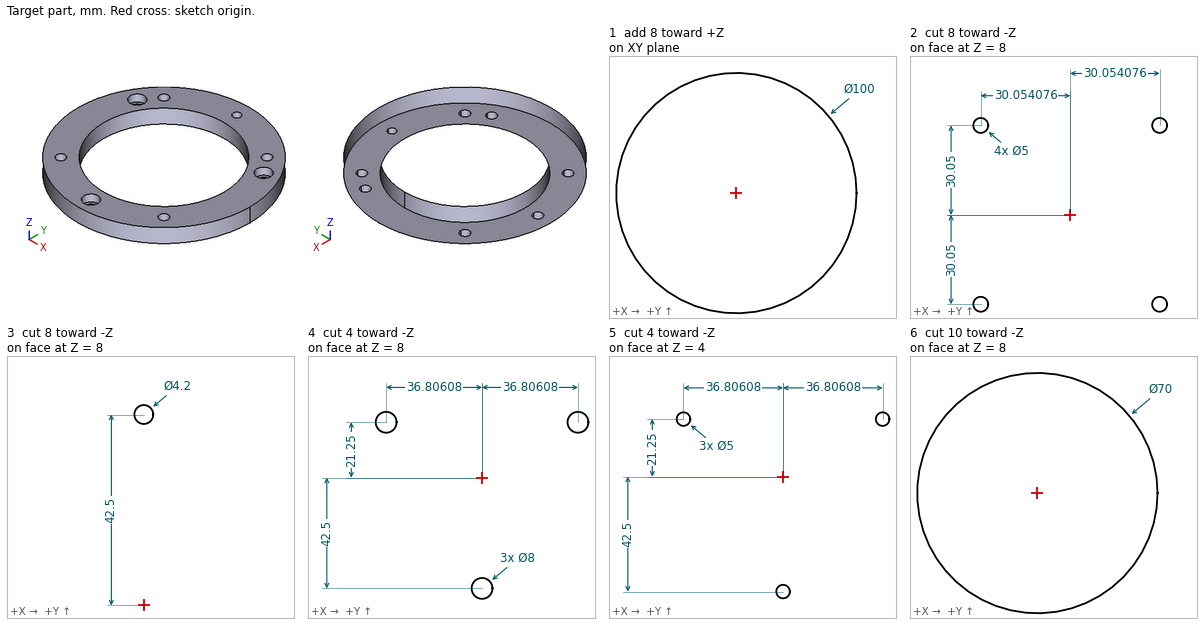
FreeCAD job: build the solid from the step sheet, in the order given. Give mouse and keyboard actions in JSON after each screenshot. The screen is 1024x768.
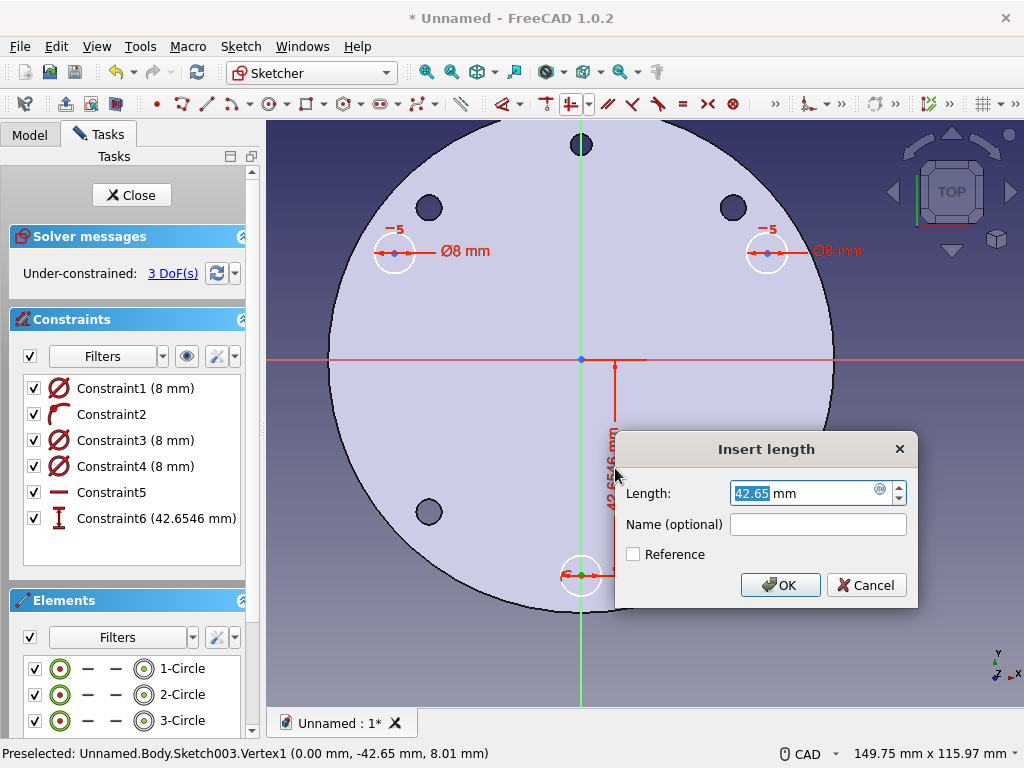
{"action": "type", "text": "42.5"}
{"action": "key", "text": "Return"}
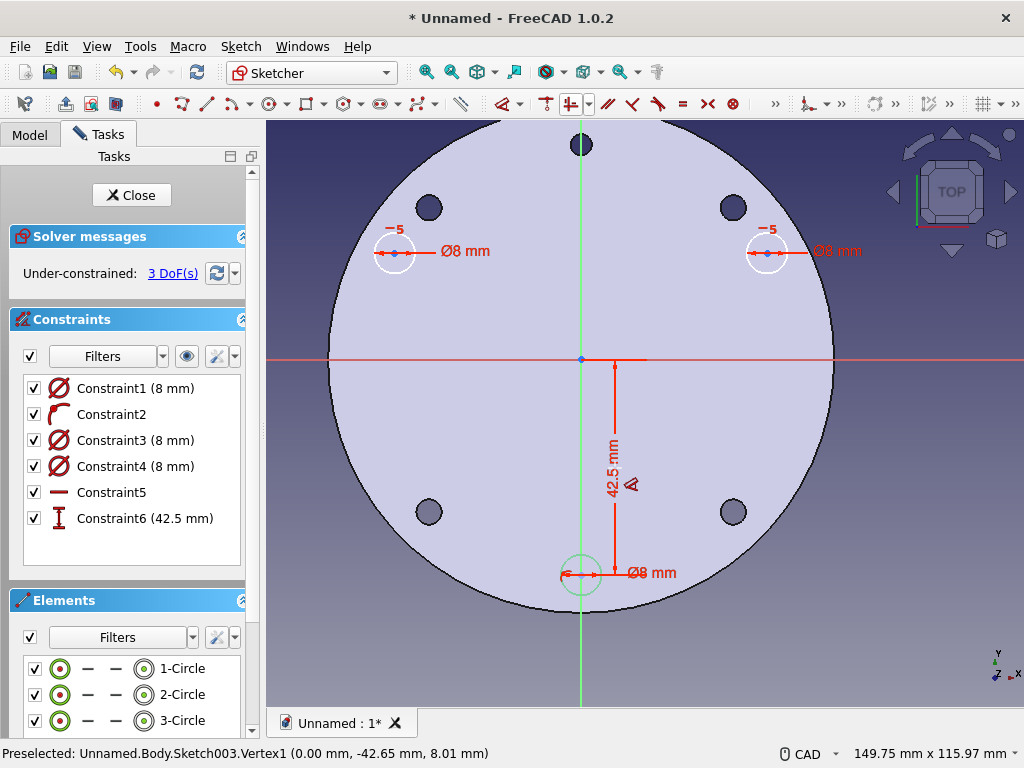
{"action": "left_click", "coordinate": [395, 253]}
{"action": "left_click", "coordinate": [361, 307]}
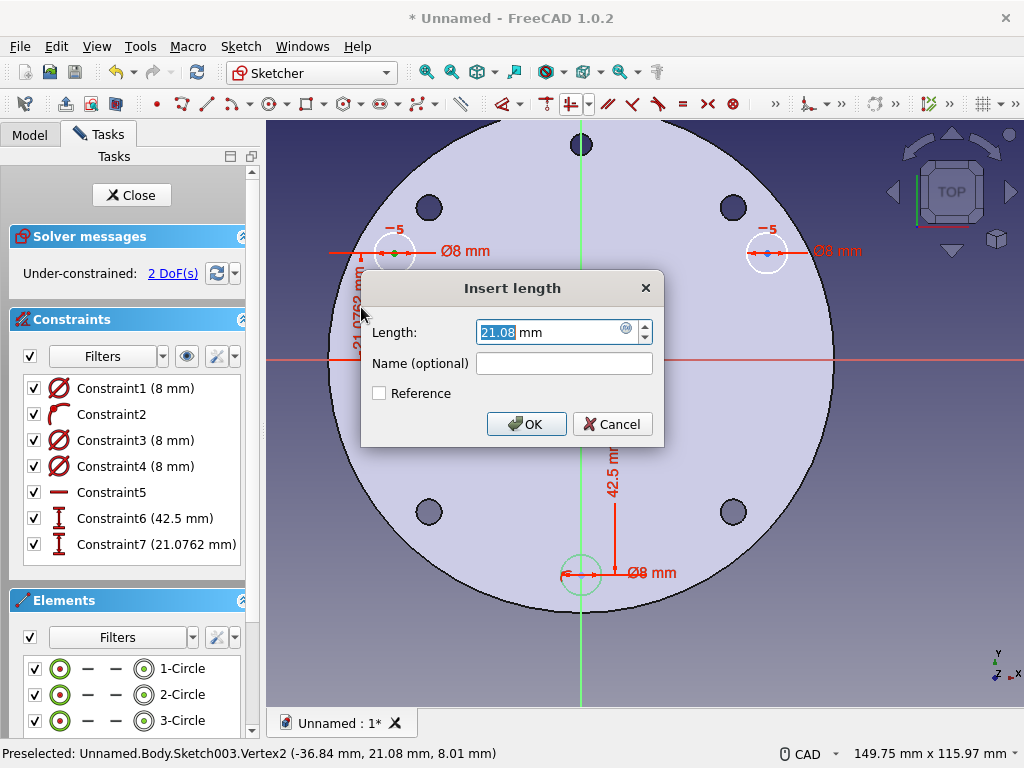
{"action": "type", "text": "21.25"}
{"action": "key", "text": "Return"}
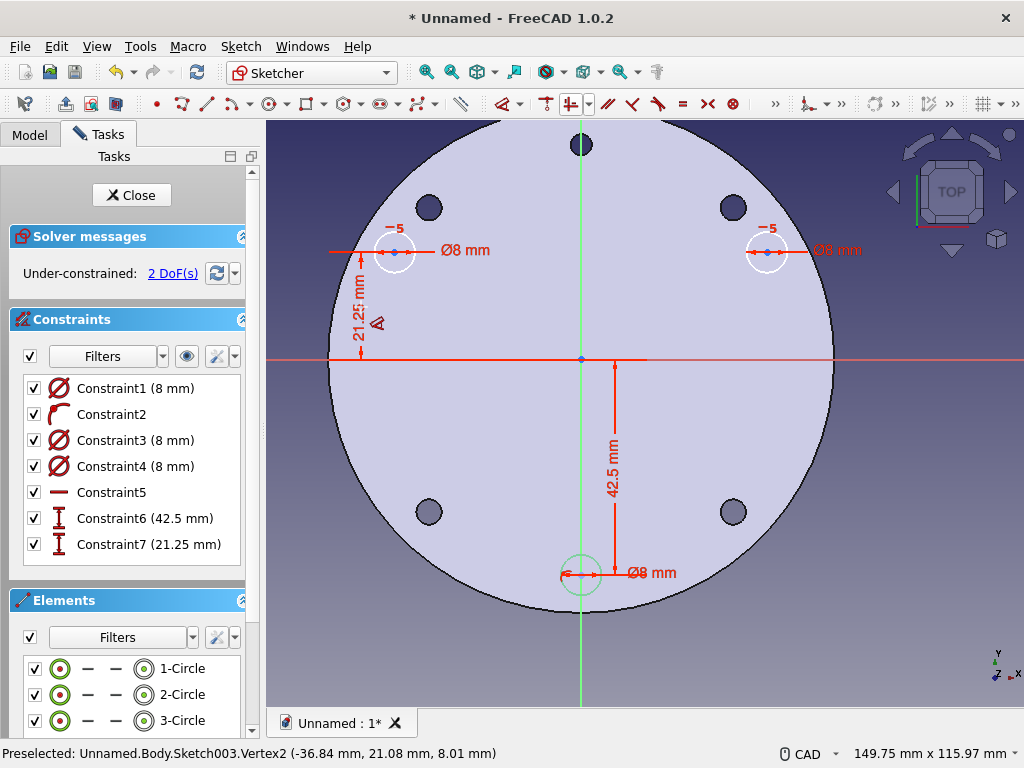
{"action": "left_click", "coordinate": [395, 252]}
{"action": "left_click", "coordinate": [488, 218]}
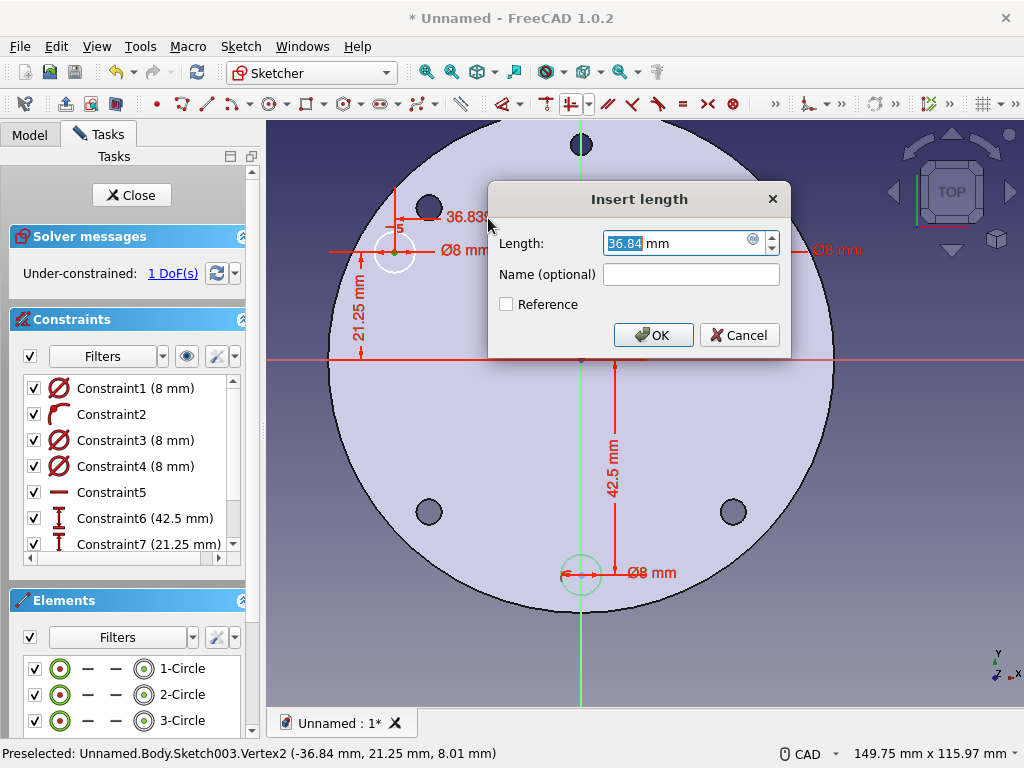
{"action": "type", "text": "36.80608"}
{"action": "key", "text": "Return"}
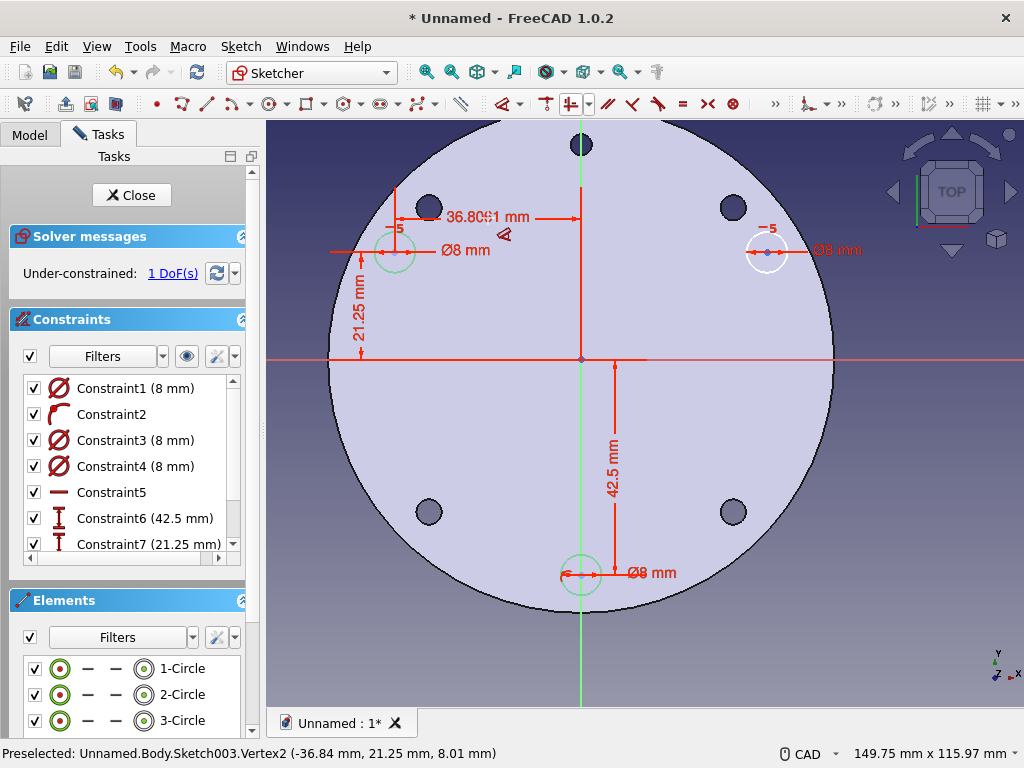
{"action": "left_click", "coordinate": [767, 252]}
{"action": "left_click", "coordinate": [674, 218]}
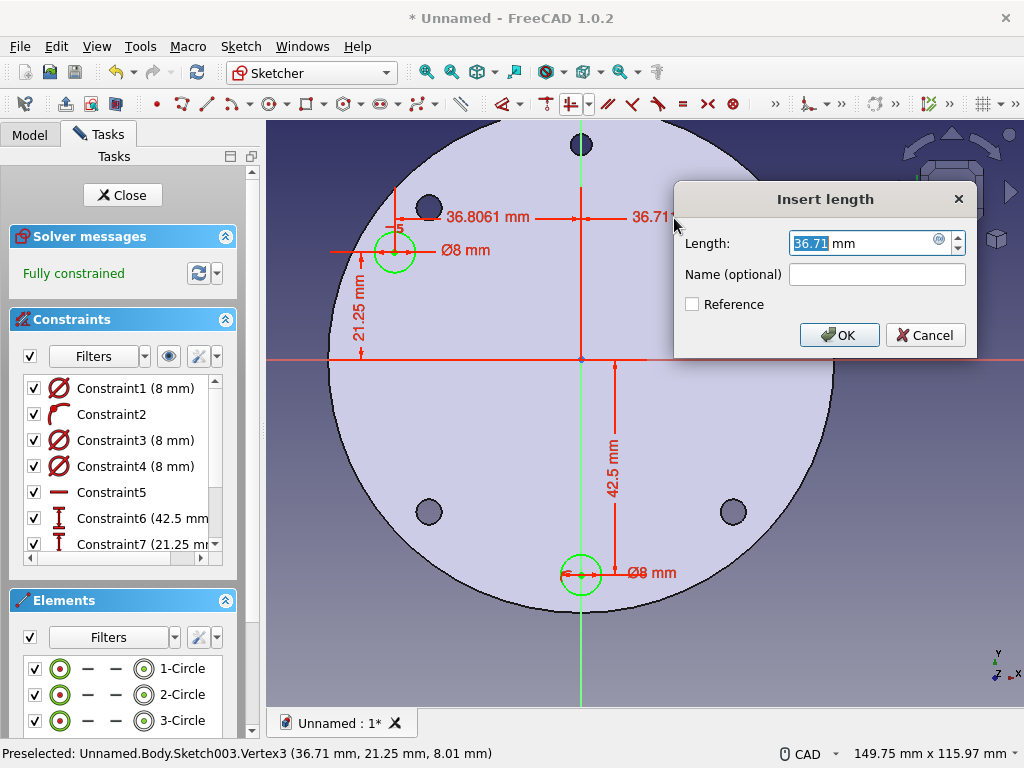
{"action": "type", "text": "36.80608"}
{"action": "key", "text": "Return"}
{"action": "key", "text": "Escape"}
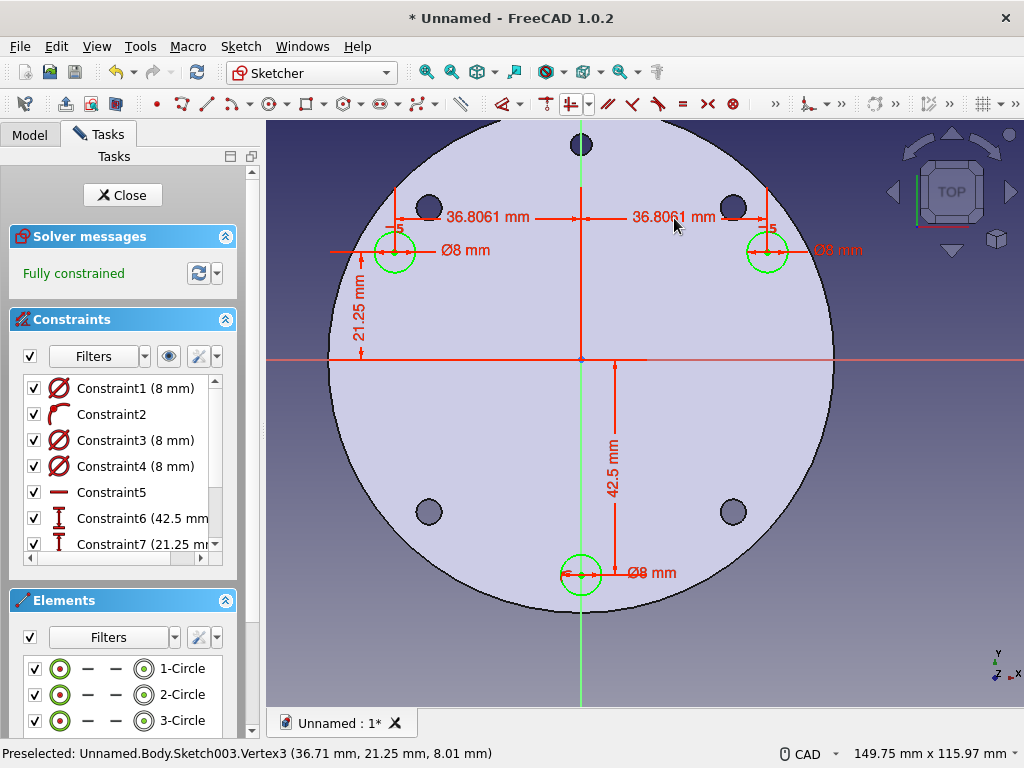
{"action": "left_click", "coordinate": [123, 195]}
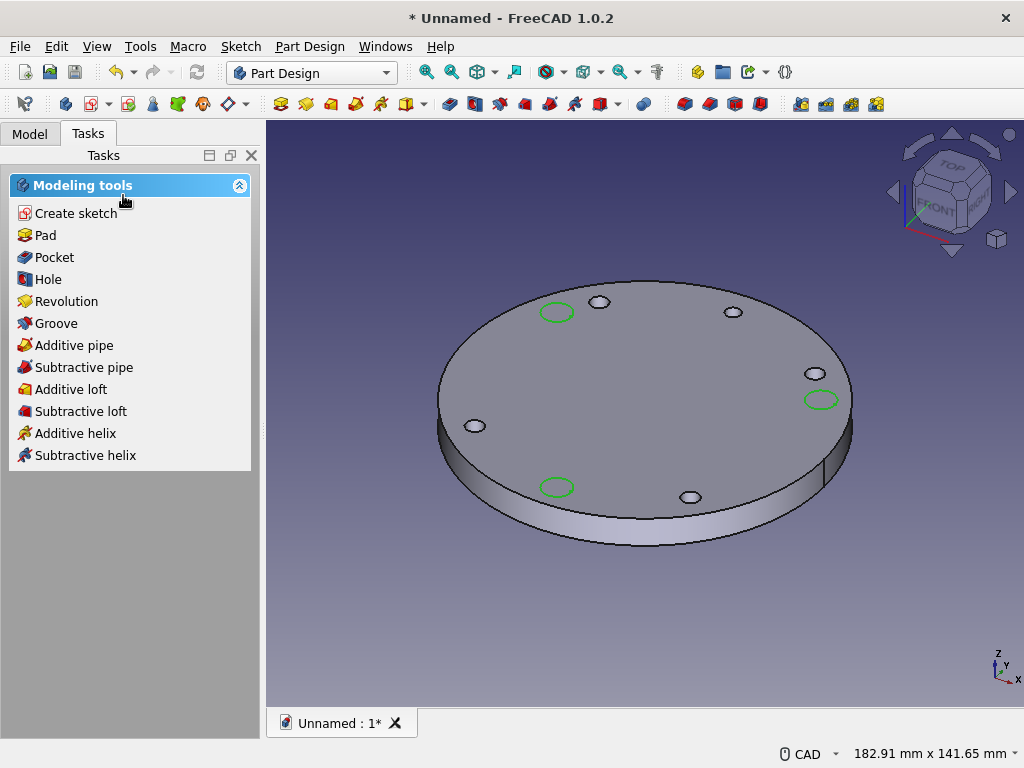
{"action": "left_click", "coordinate": [450, 104]}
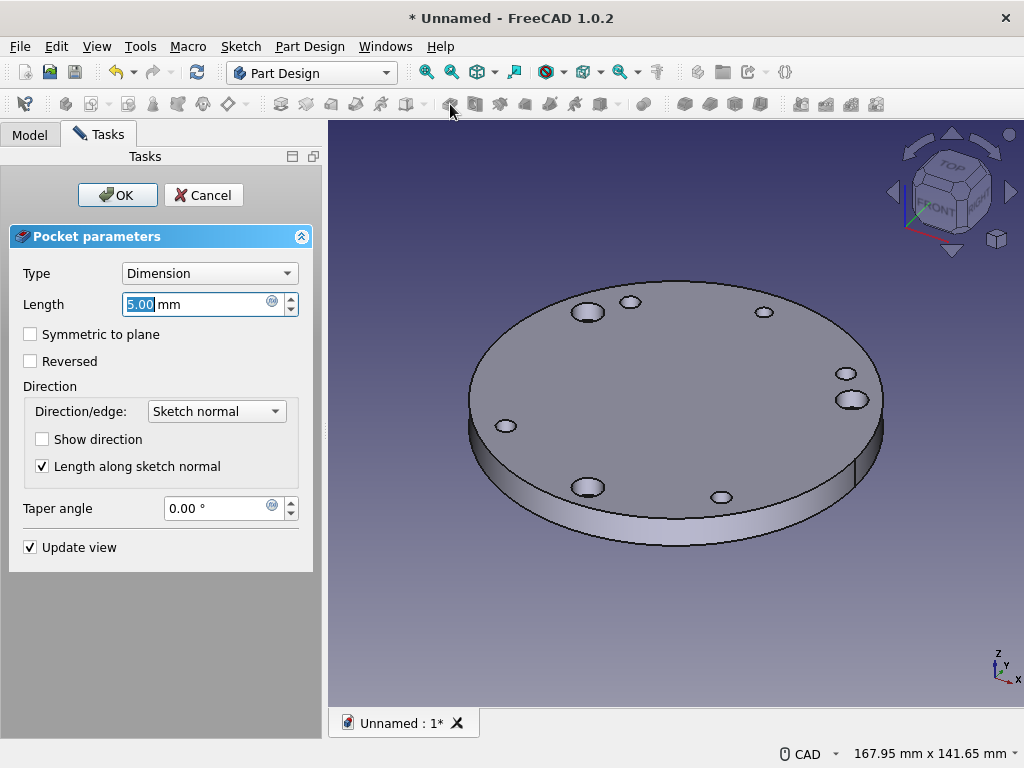
{"action": "type", "text": "4"}
{"action": "key", "text": "Tab"}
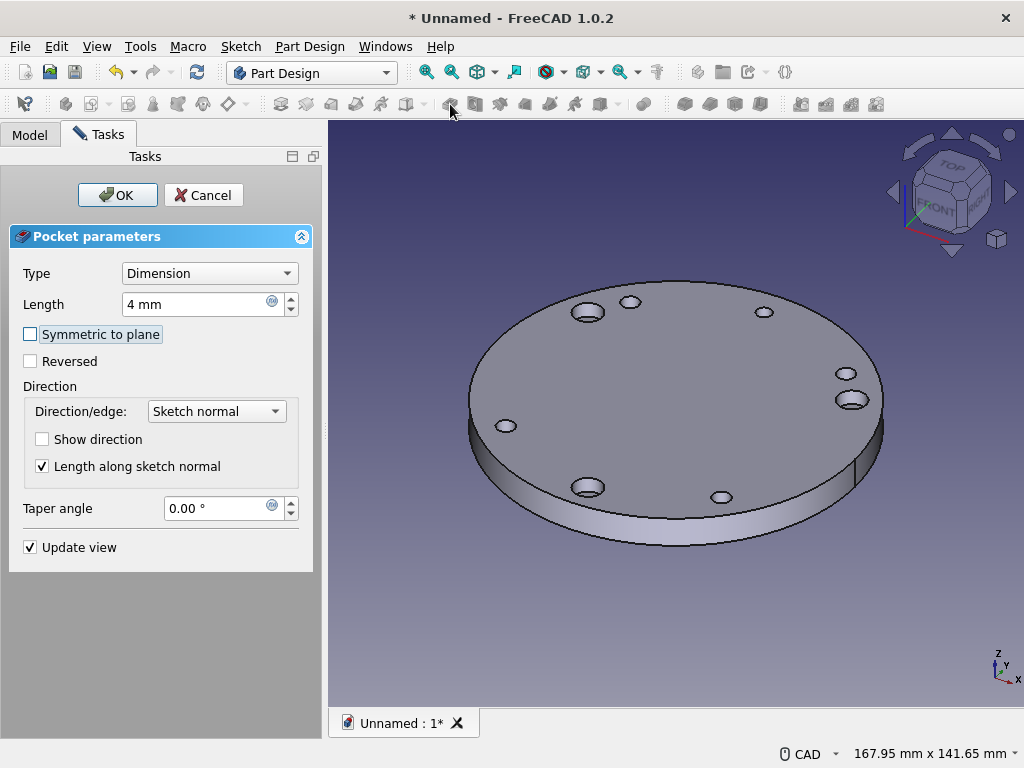
{"action": "left_click", "coordinate": [118, 195]}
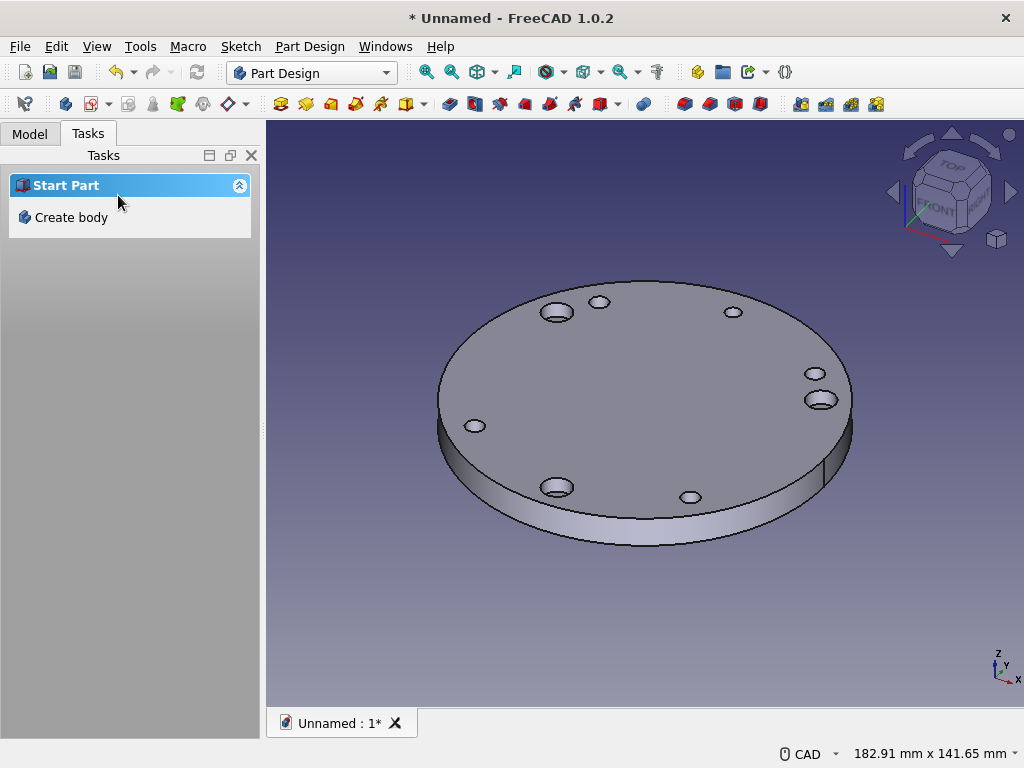
{"action": "key", "text": "0"}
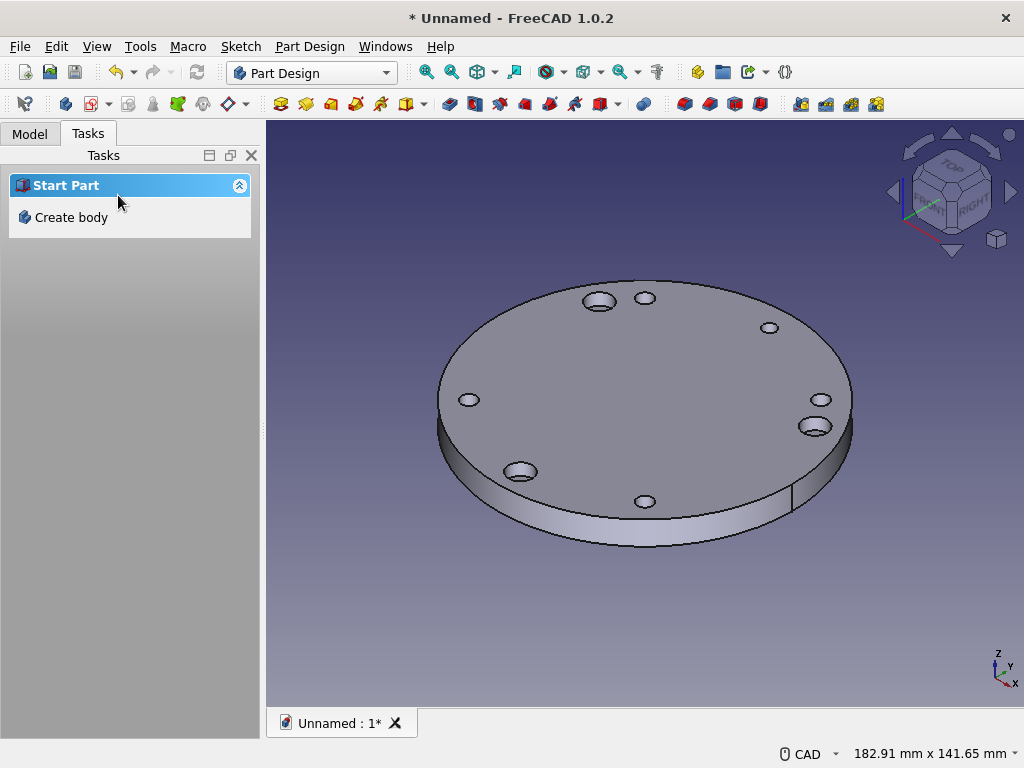
{"action": "key", "text": "2"}